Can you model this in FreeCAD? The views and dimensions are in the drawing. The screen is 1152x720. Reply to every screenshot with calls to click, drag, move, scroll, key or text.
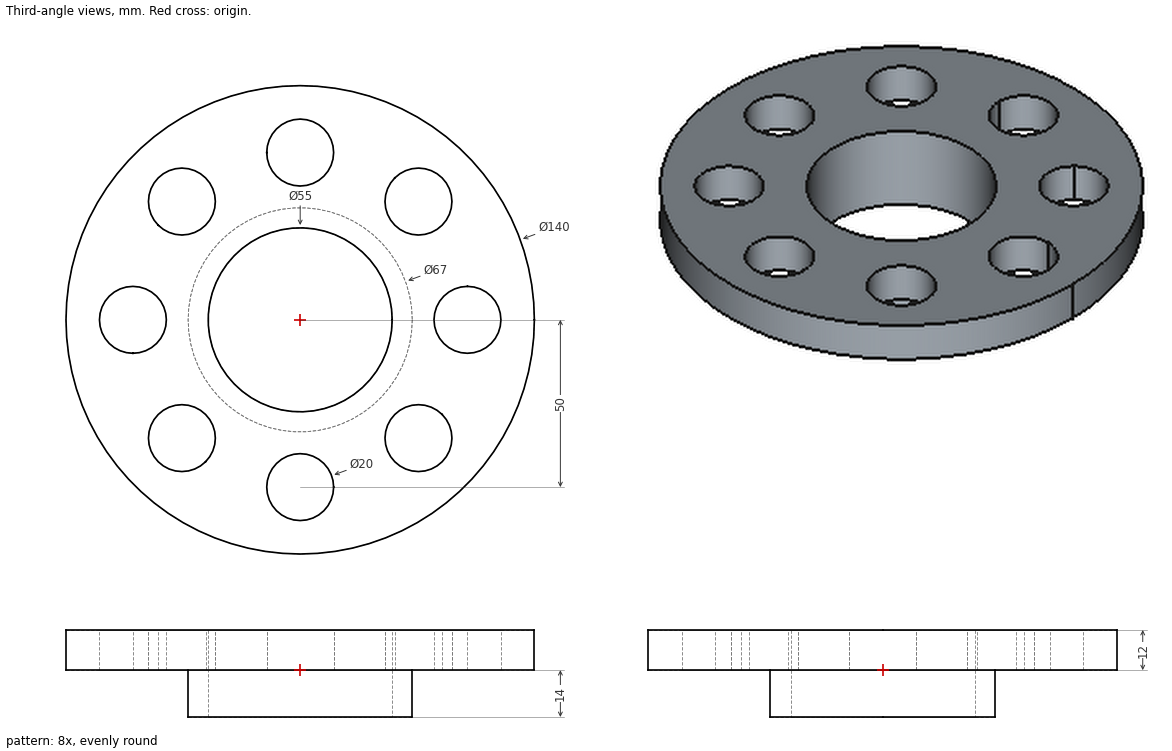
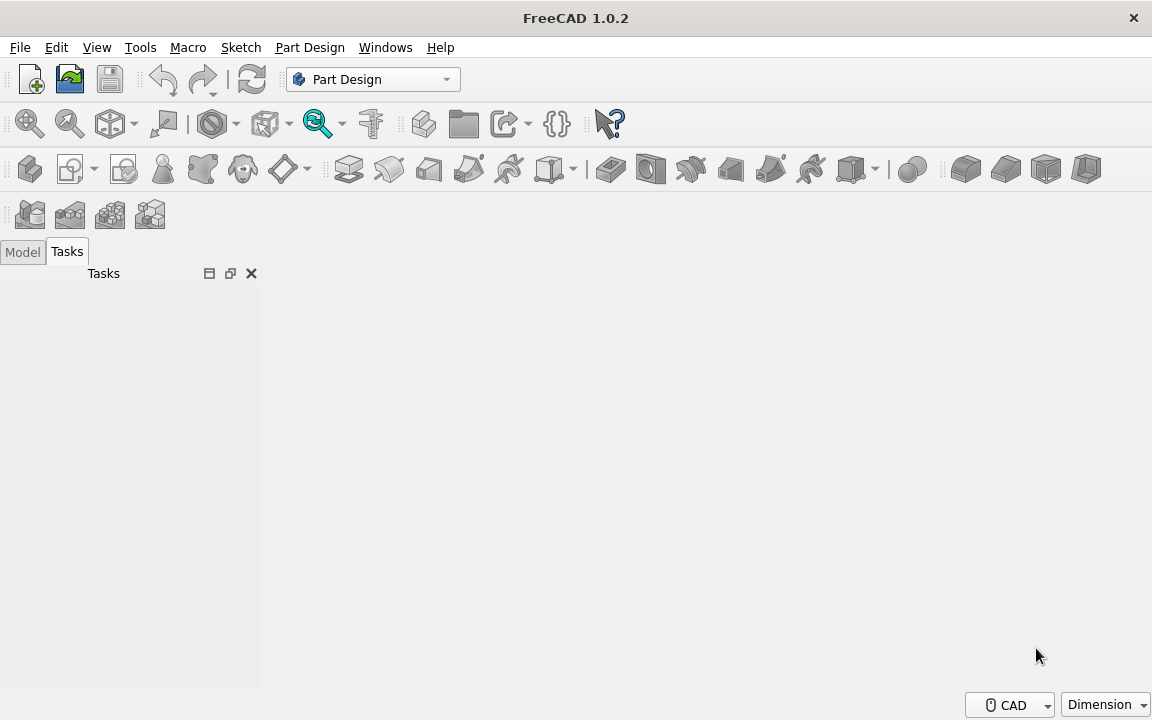
key(ctrl+n)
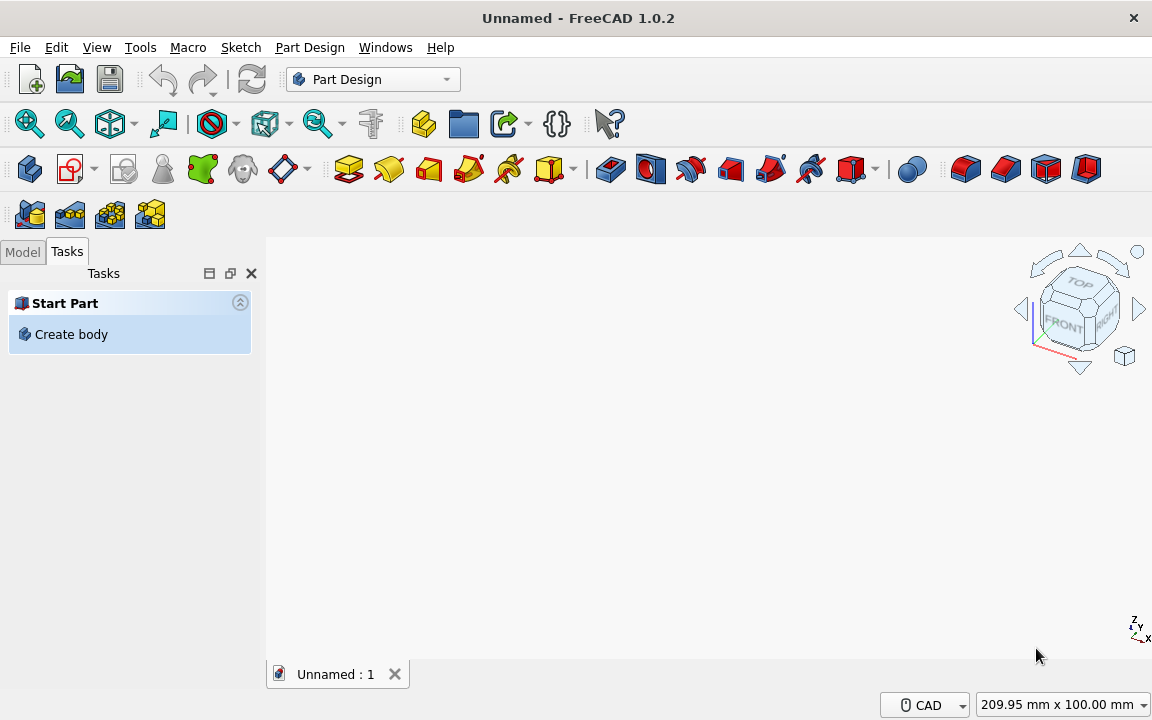
click(70, 170)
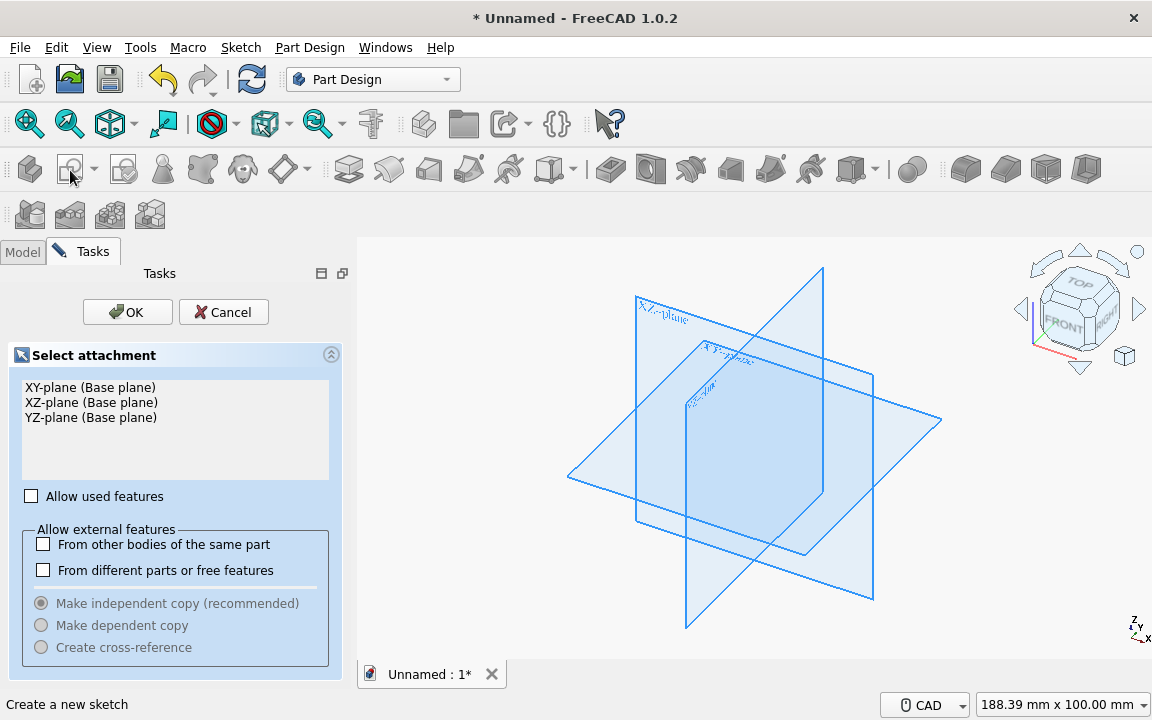
click(82, 388)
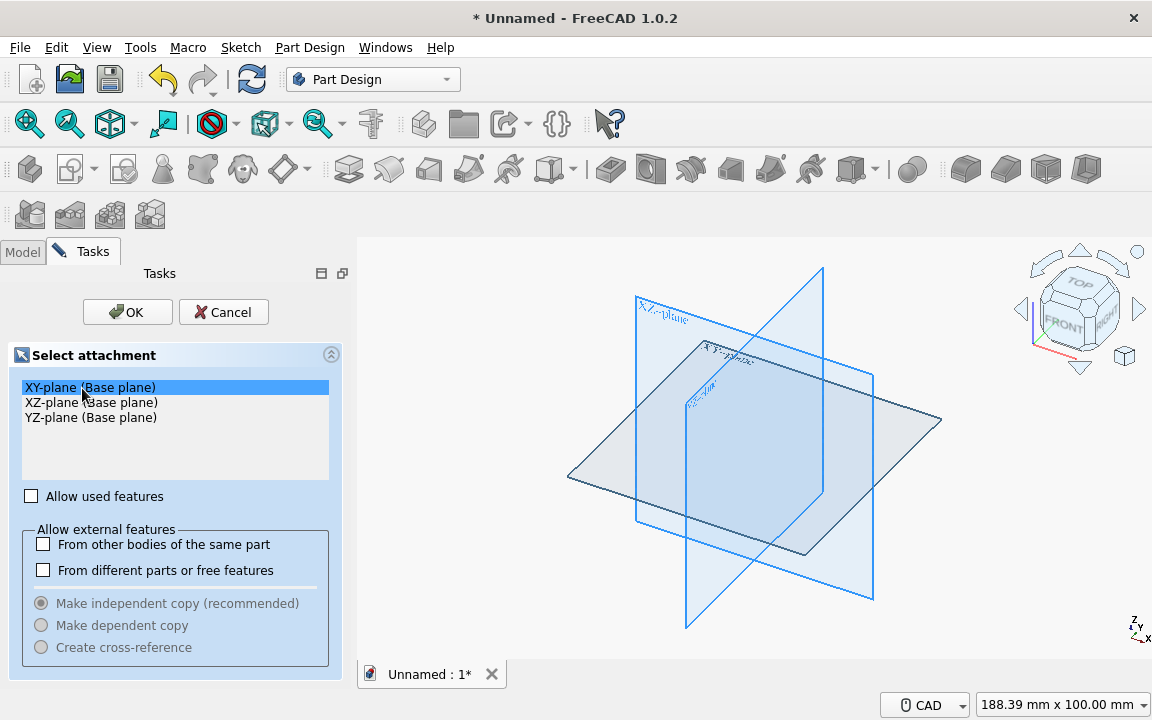
click(128, 312)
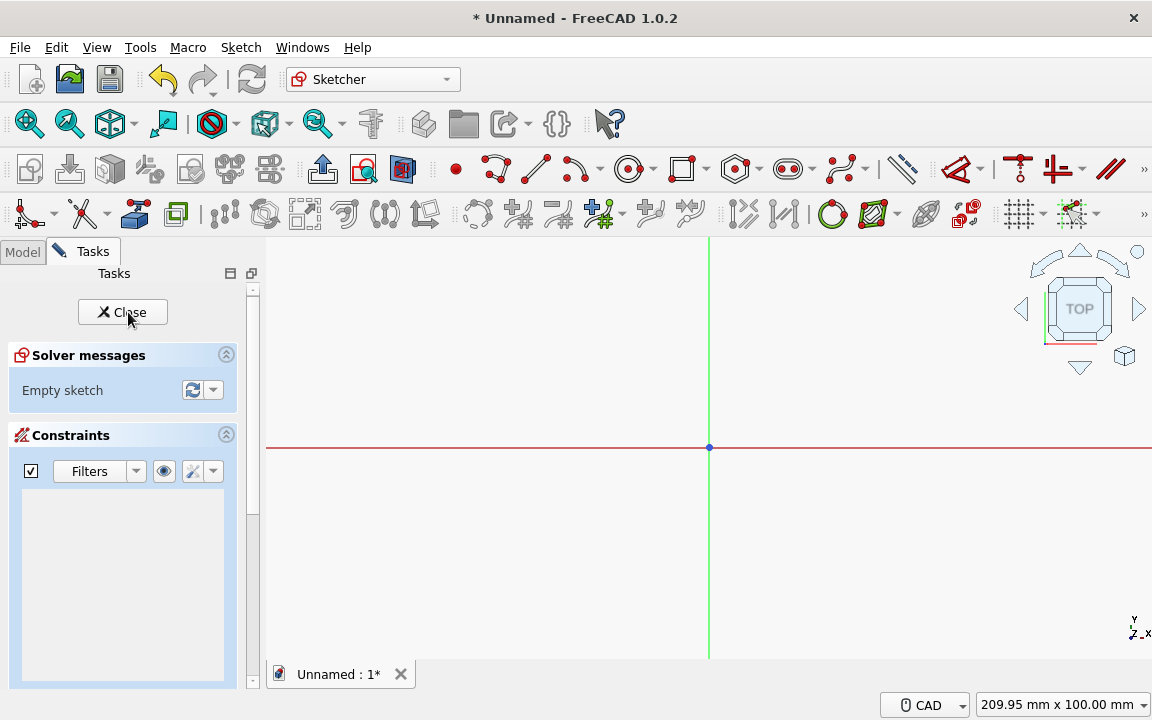
scroll(585, 448, down, 4)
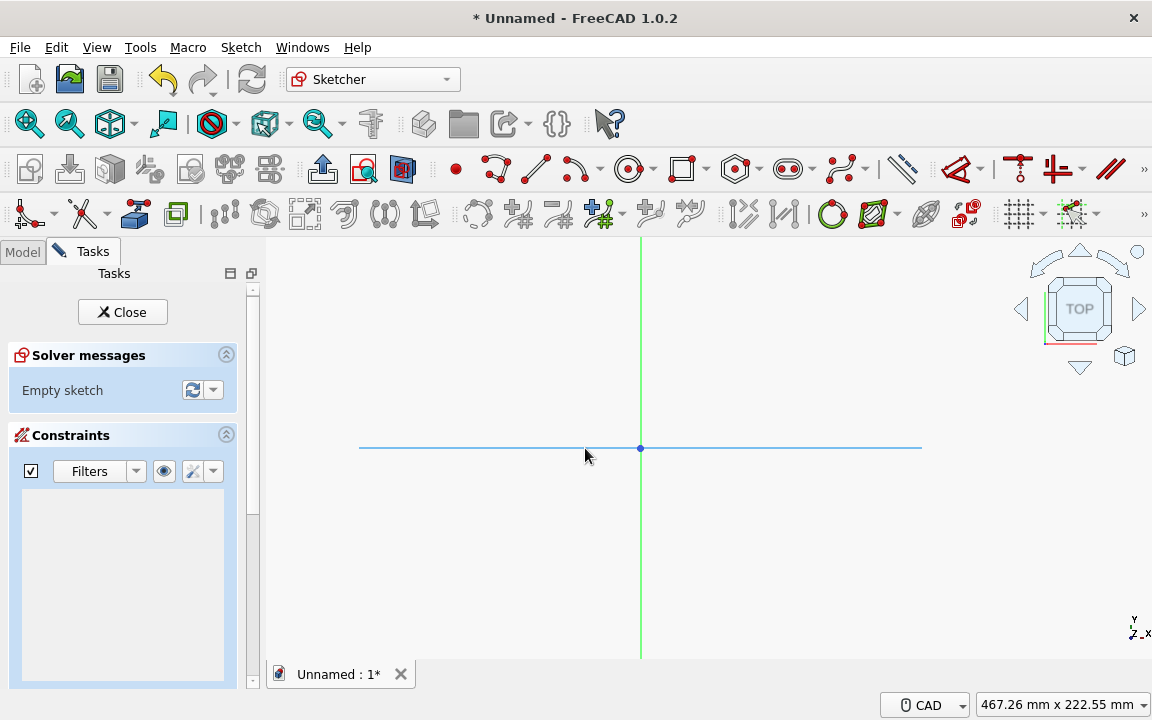
key(g)
key(c)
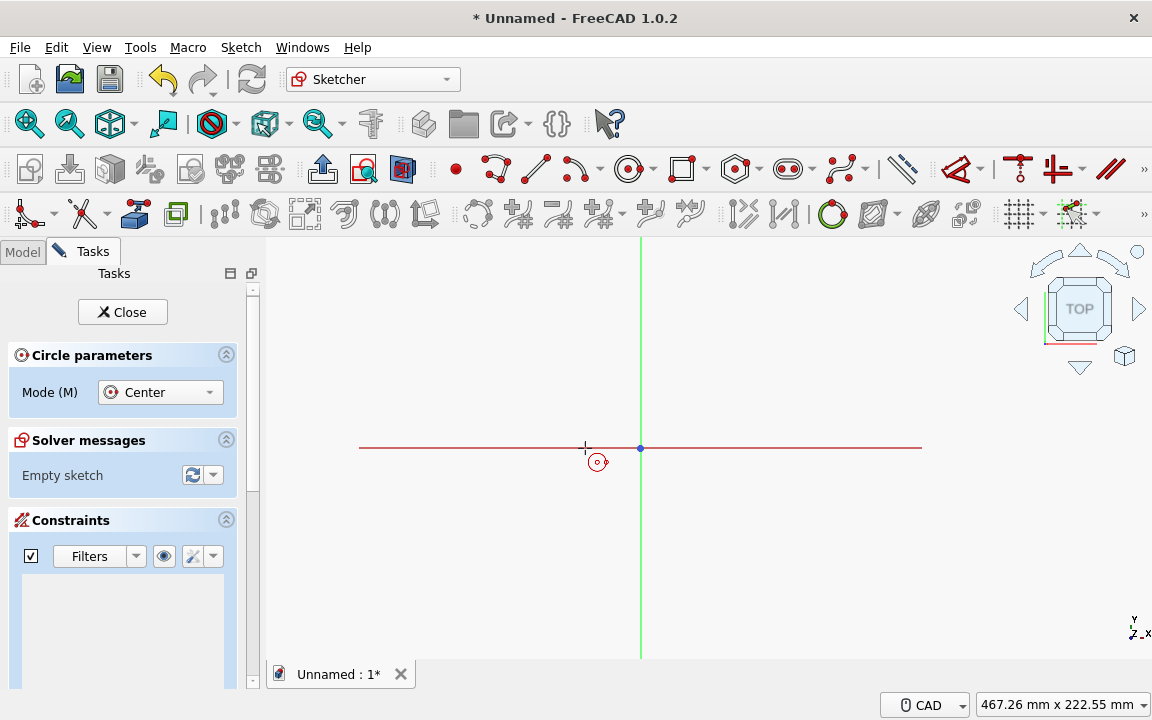
click(641, 448)
move(735, 354)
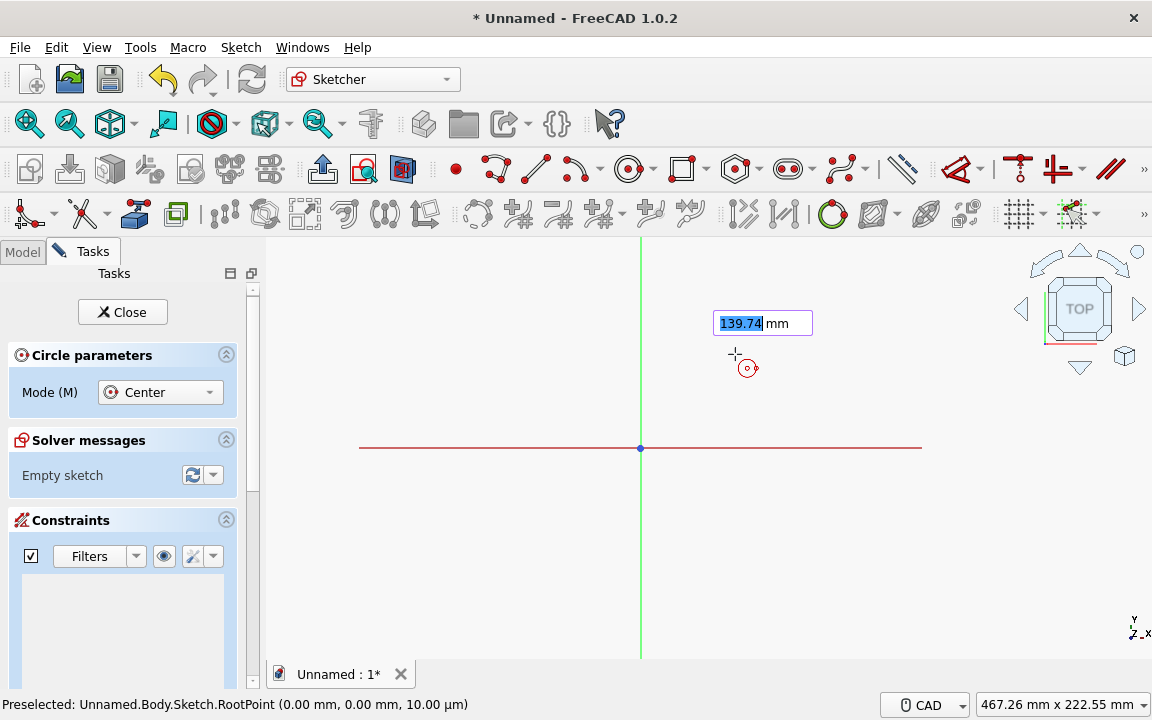
text(140)
key(Return)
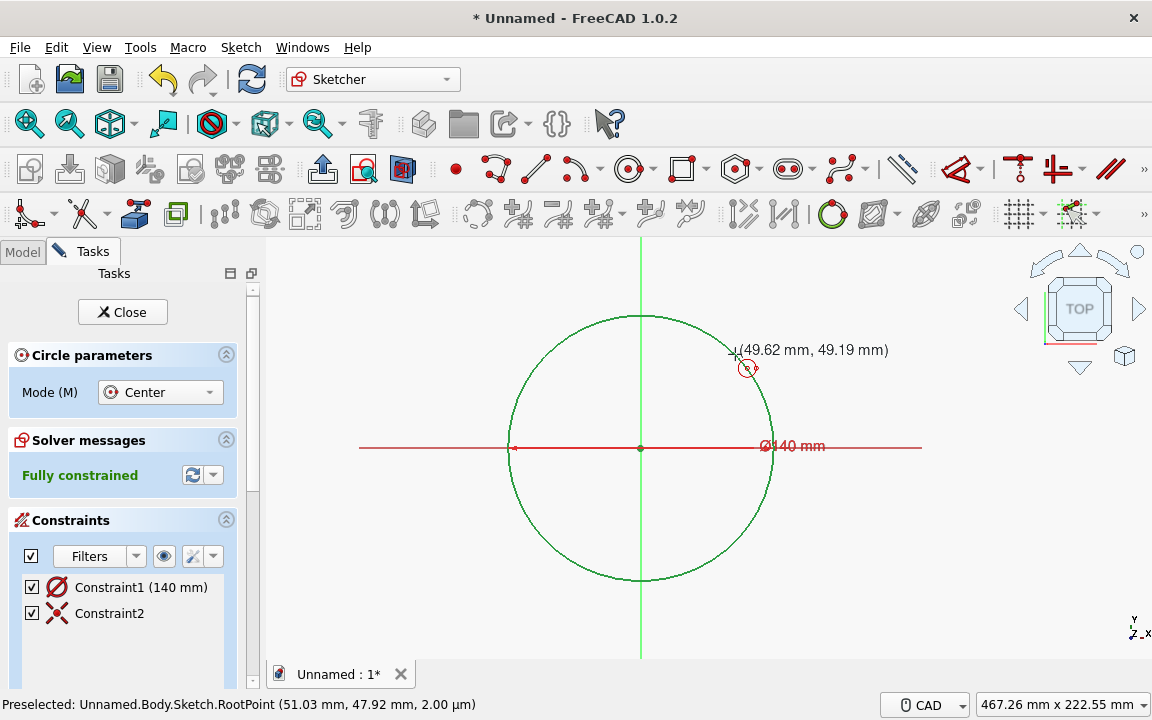
click(641, 448)
move(678, 411)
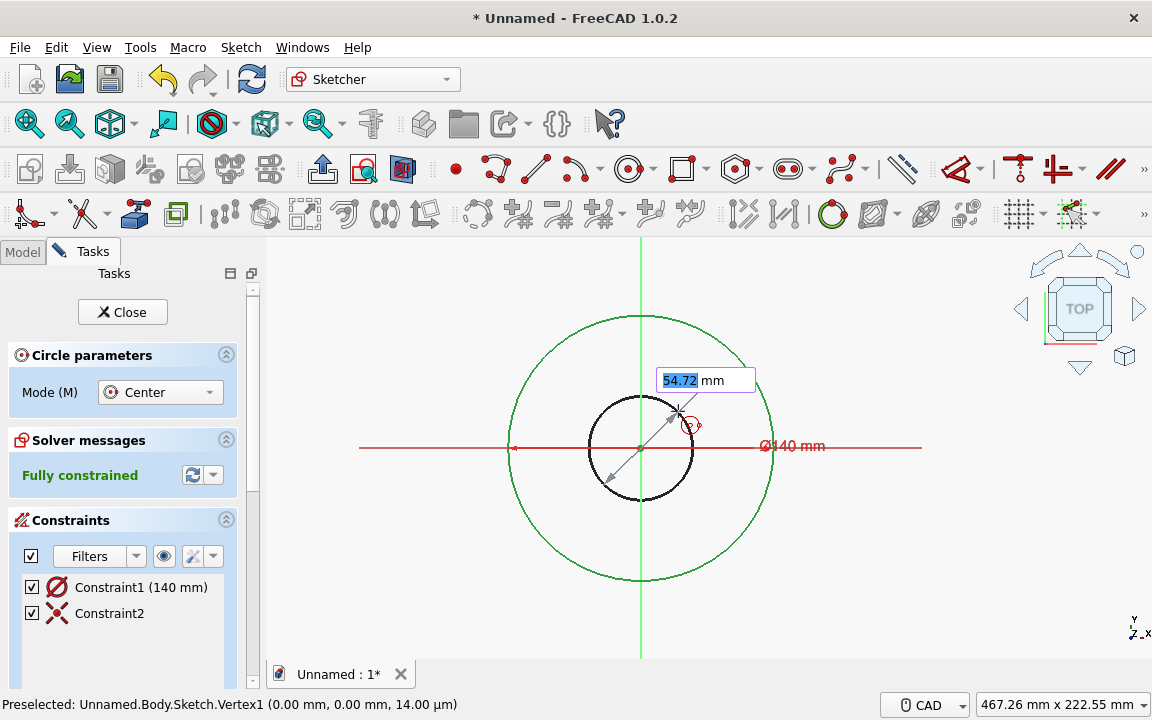
text(55)
key(Return)
key(Escape)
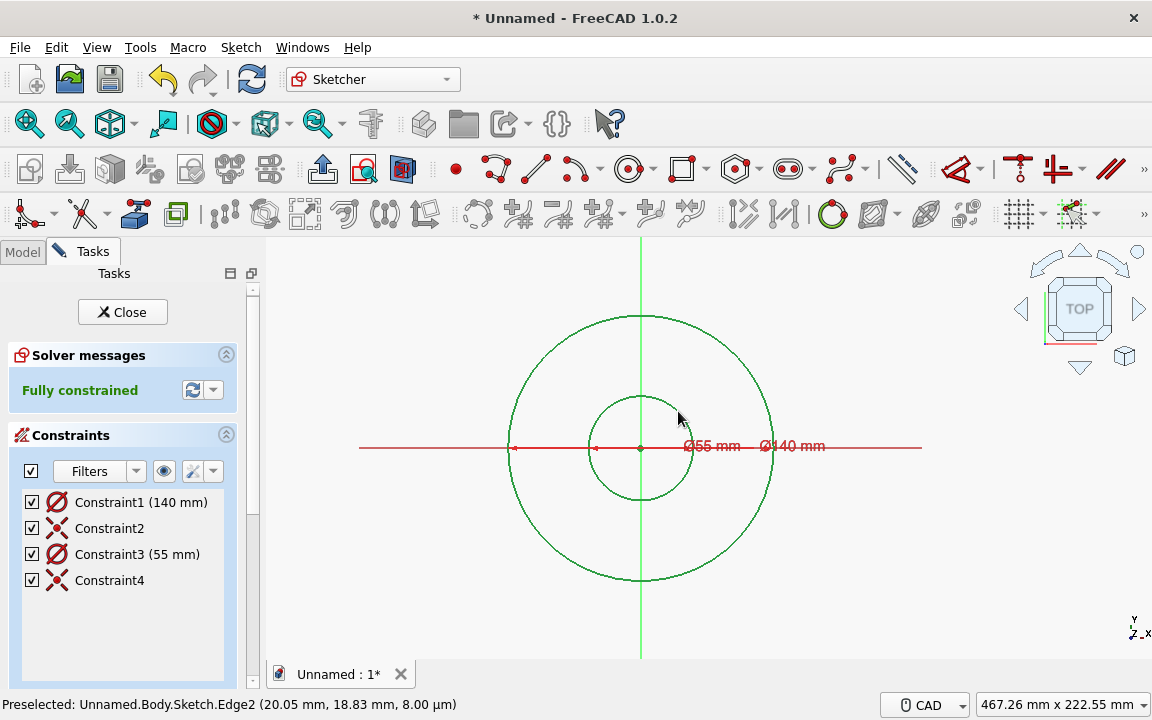
click(123, 312)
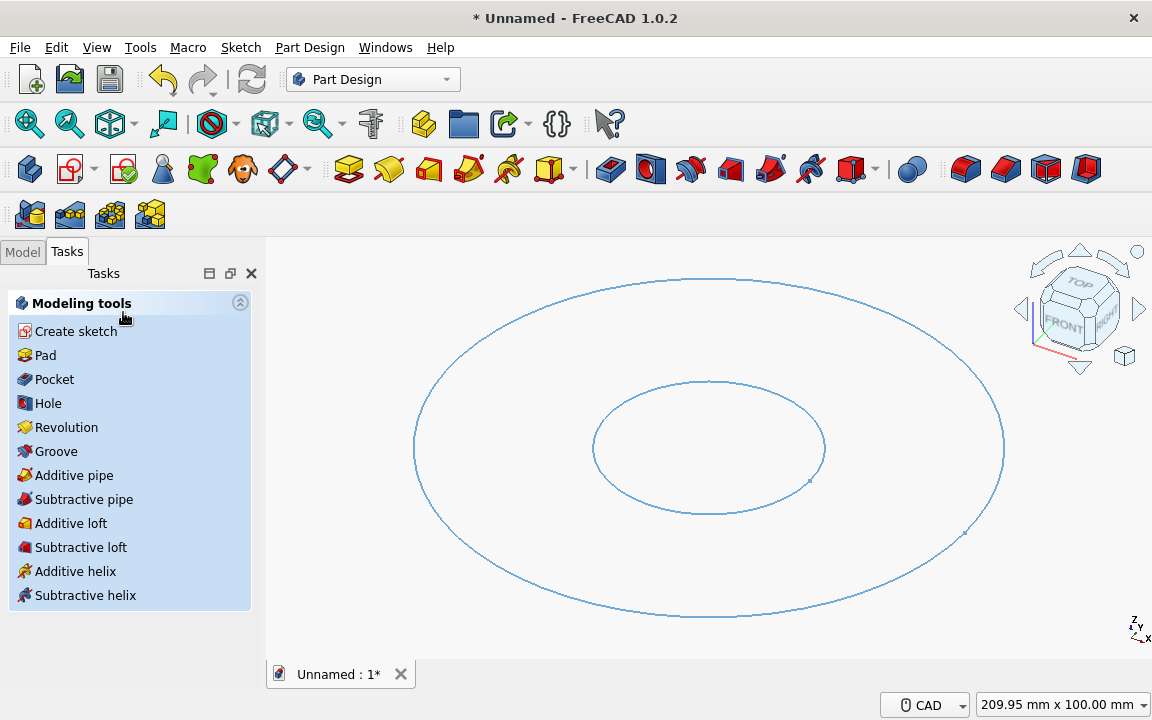
click(350, 170)